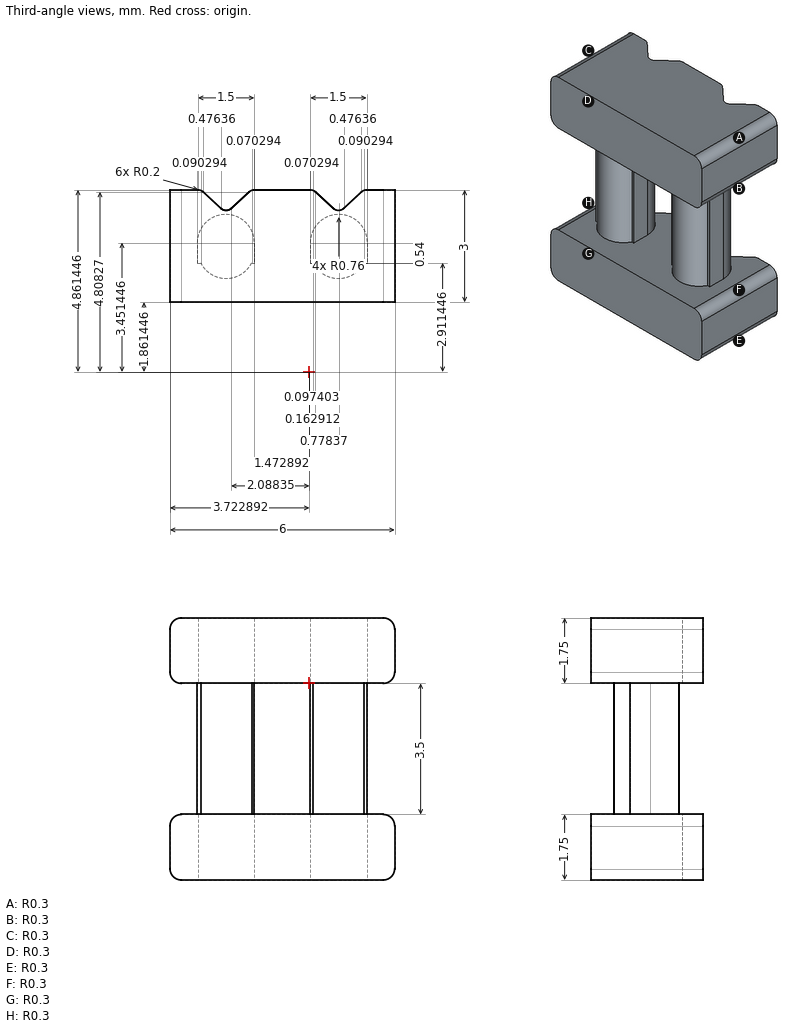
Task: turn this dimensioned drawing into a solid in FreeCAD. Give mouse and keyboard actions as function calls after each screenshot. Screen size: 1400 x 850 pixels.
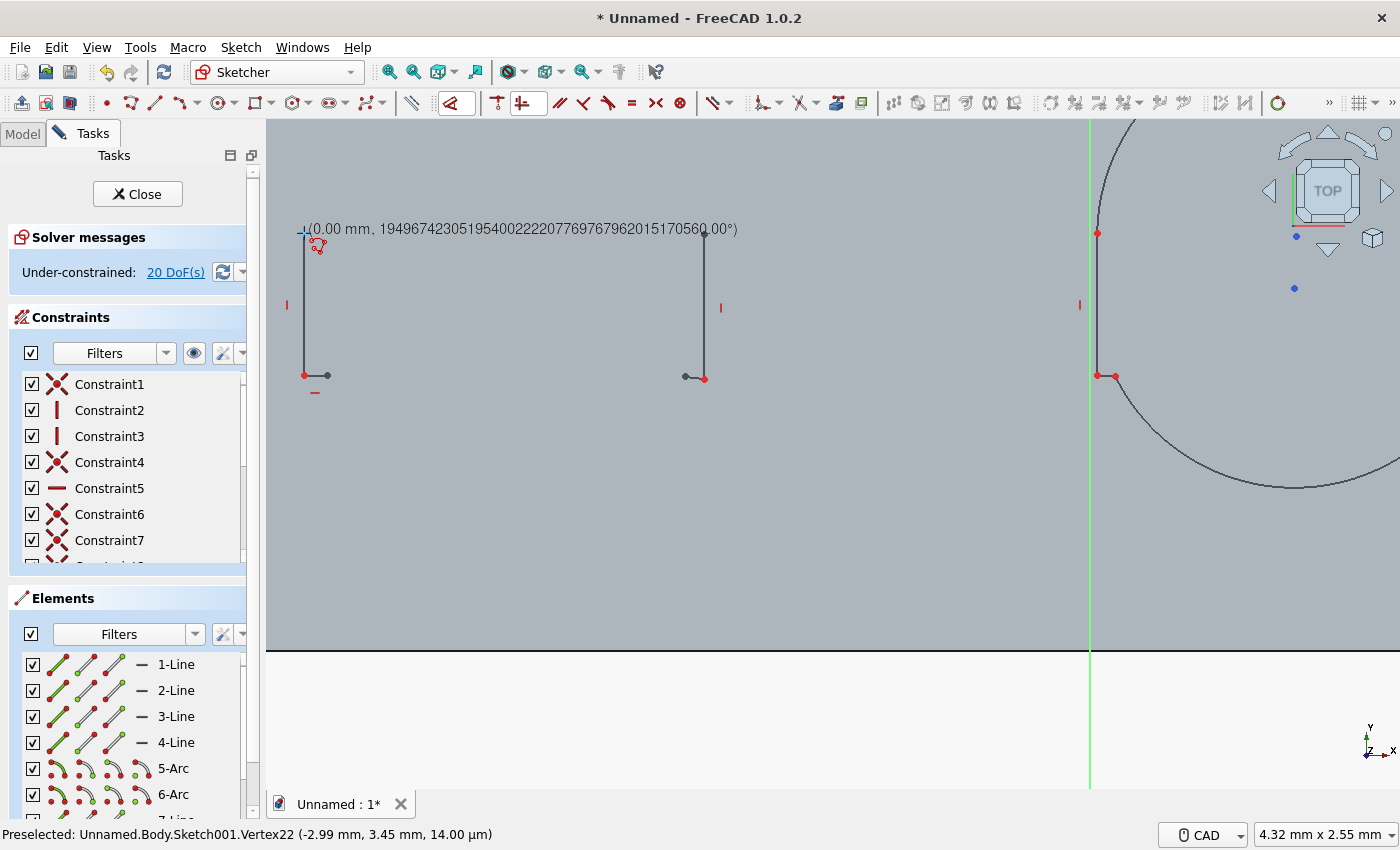
click(180, 104)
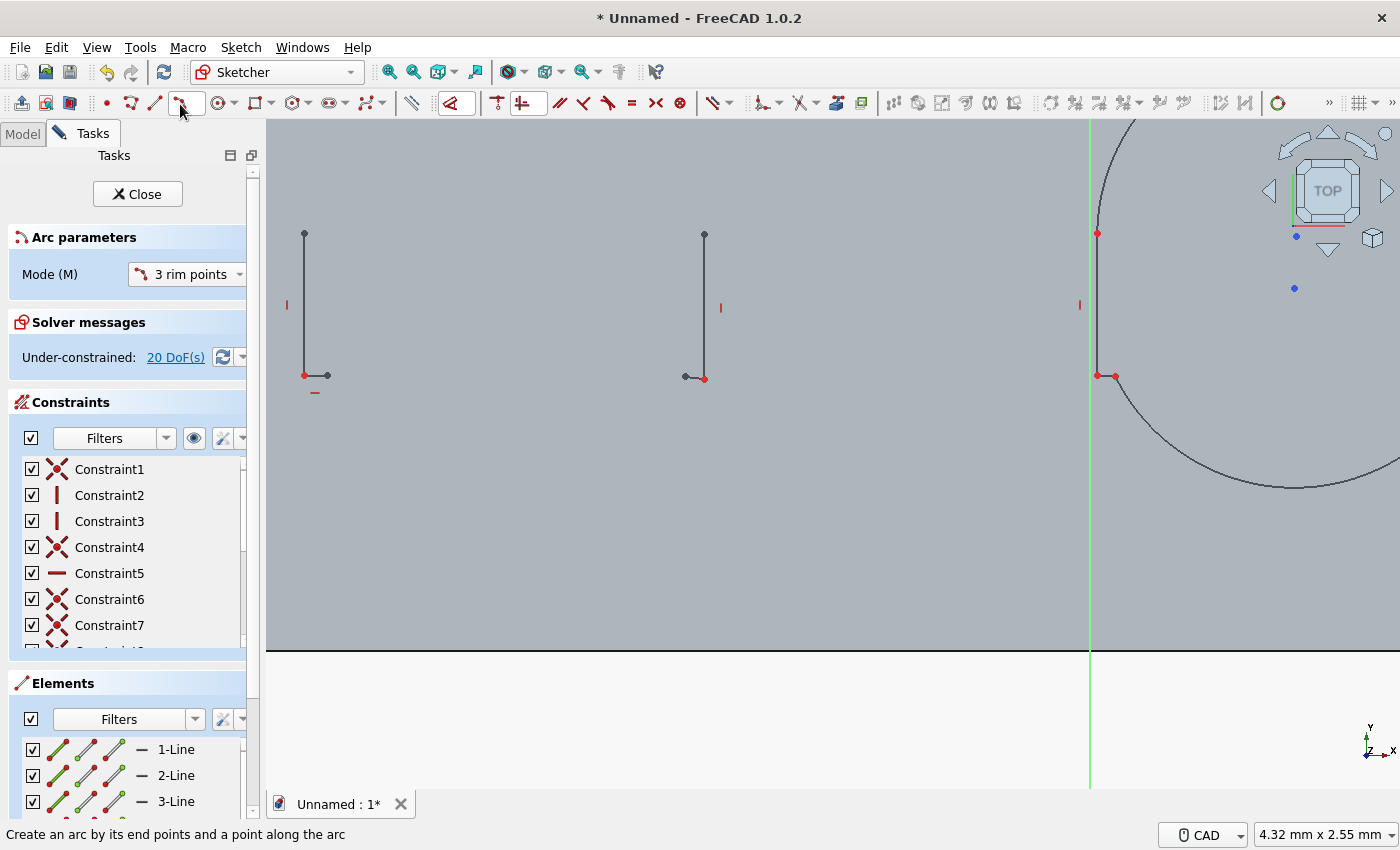
scroll(685, 375, up, 3)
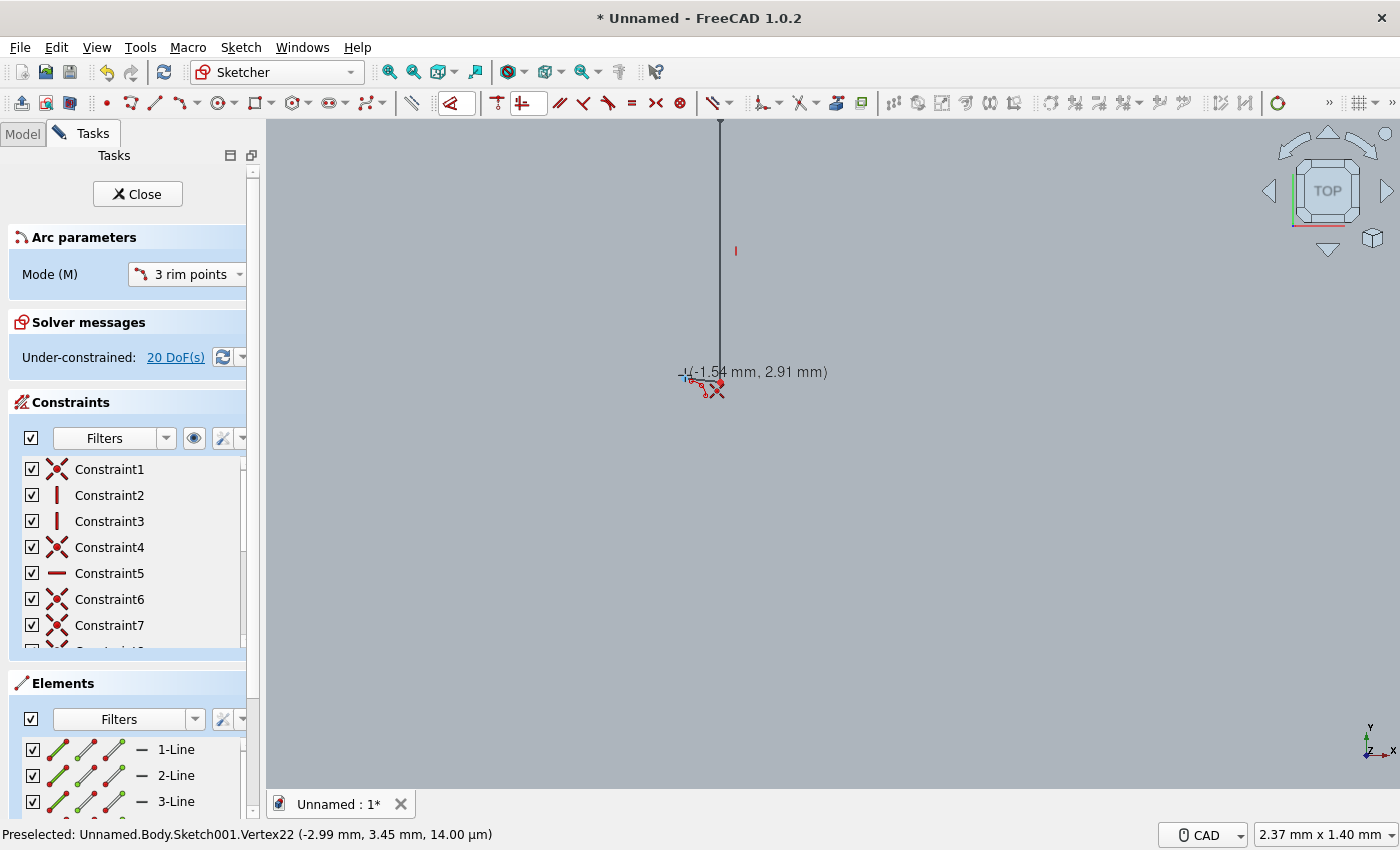
click(685, 378)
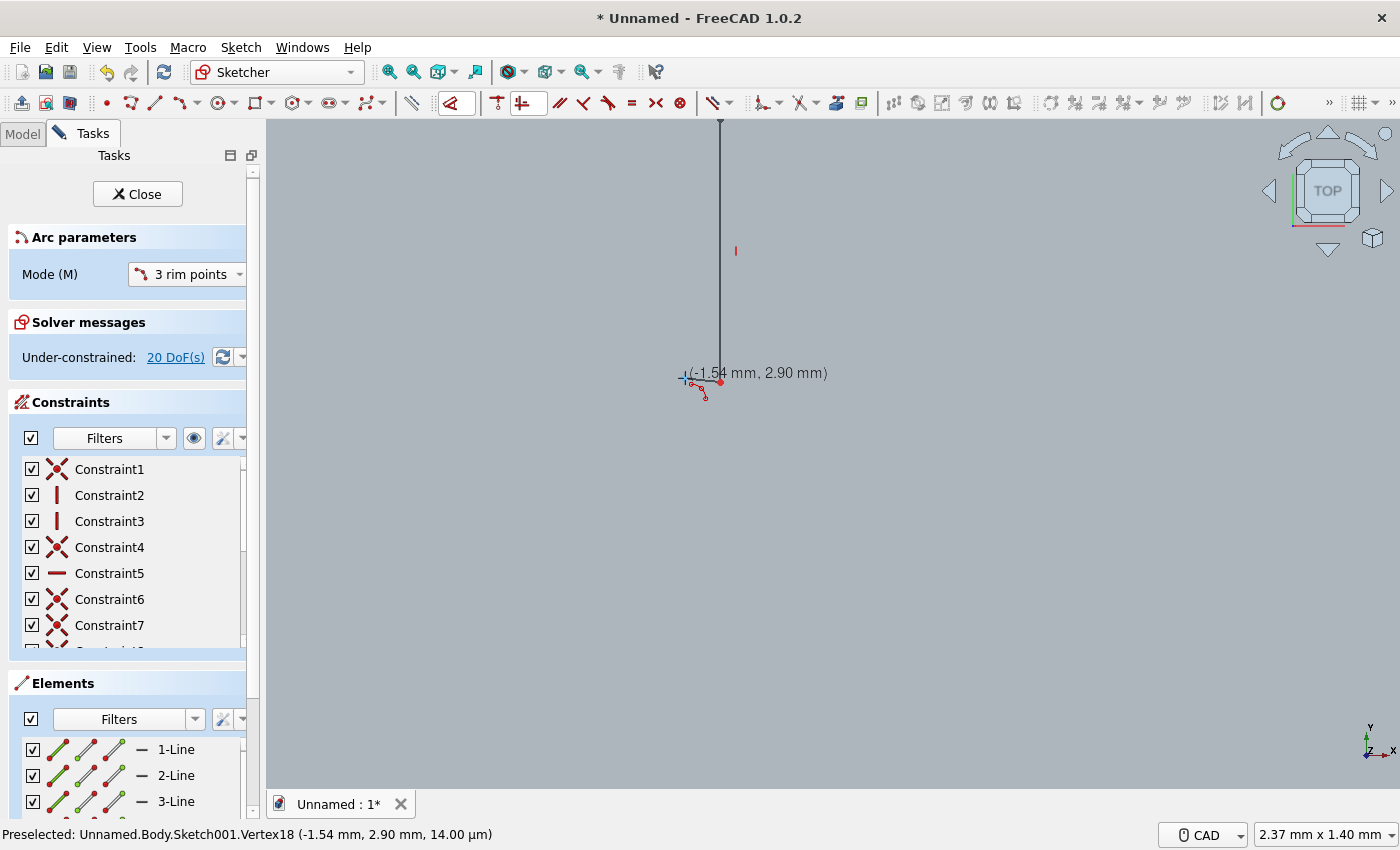
scroll(685, 376, down, 8)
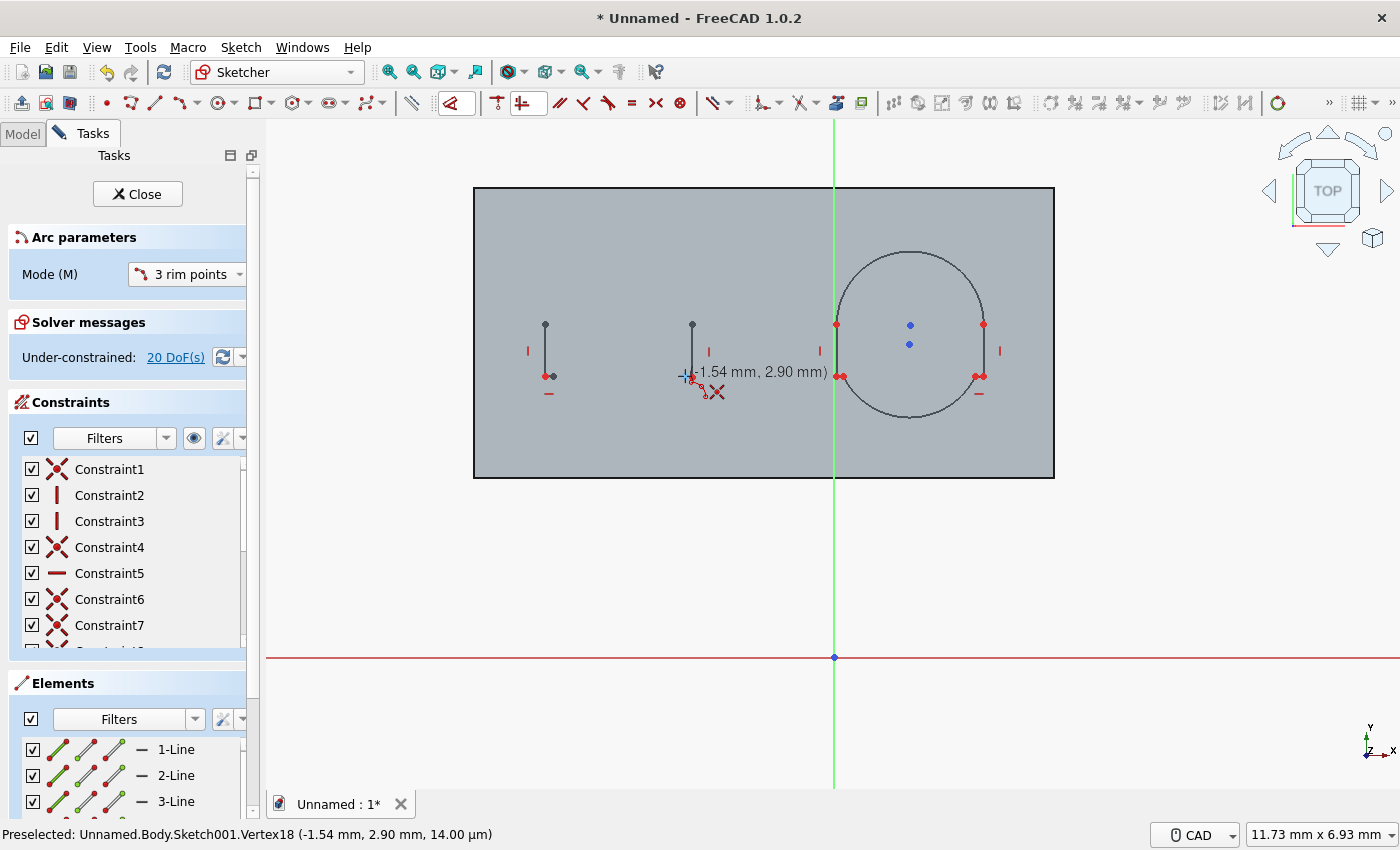
scroll(554, 376, up, 7)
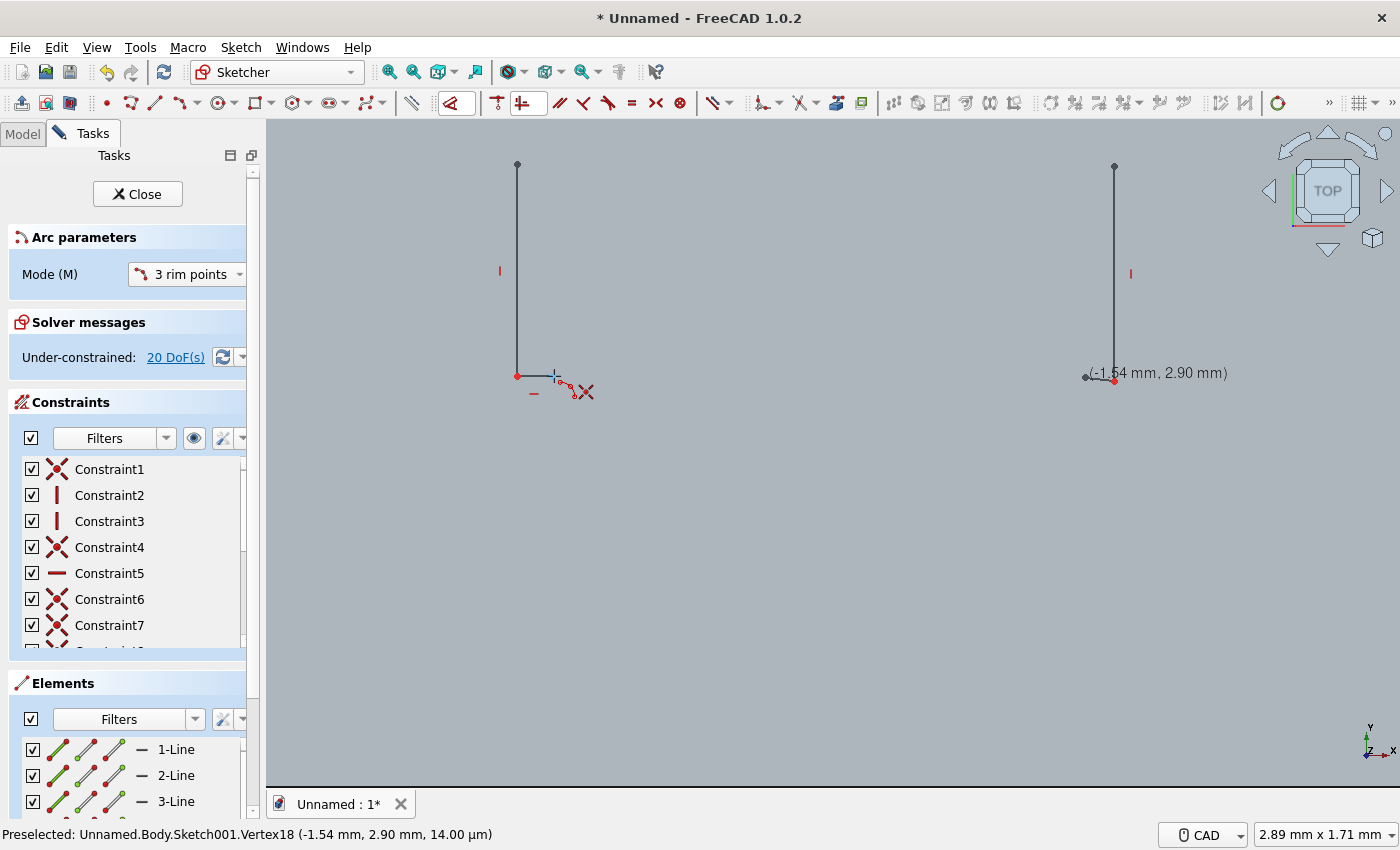
click(553, 376)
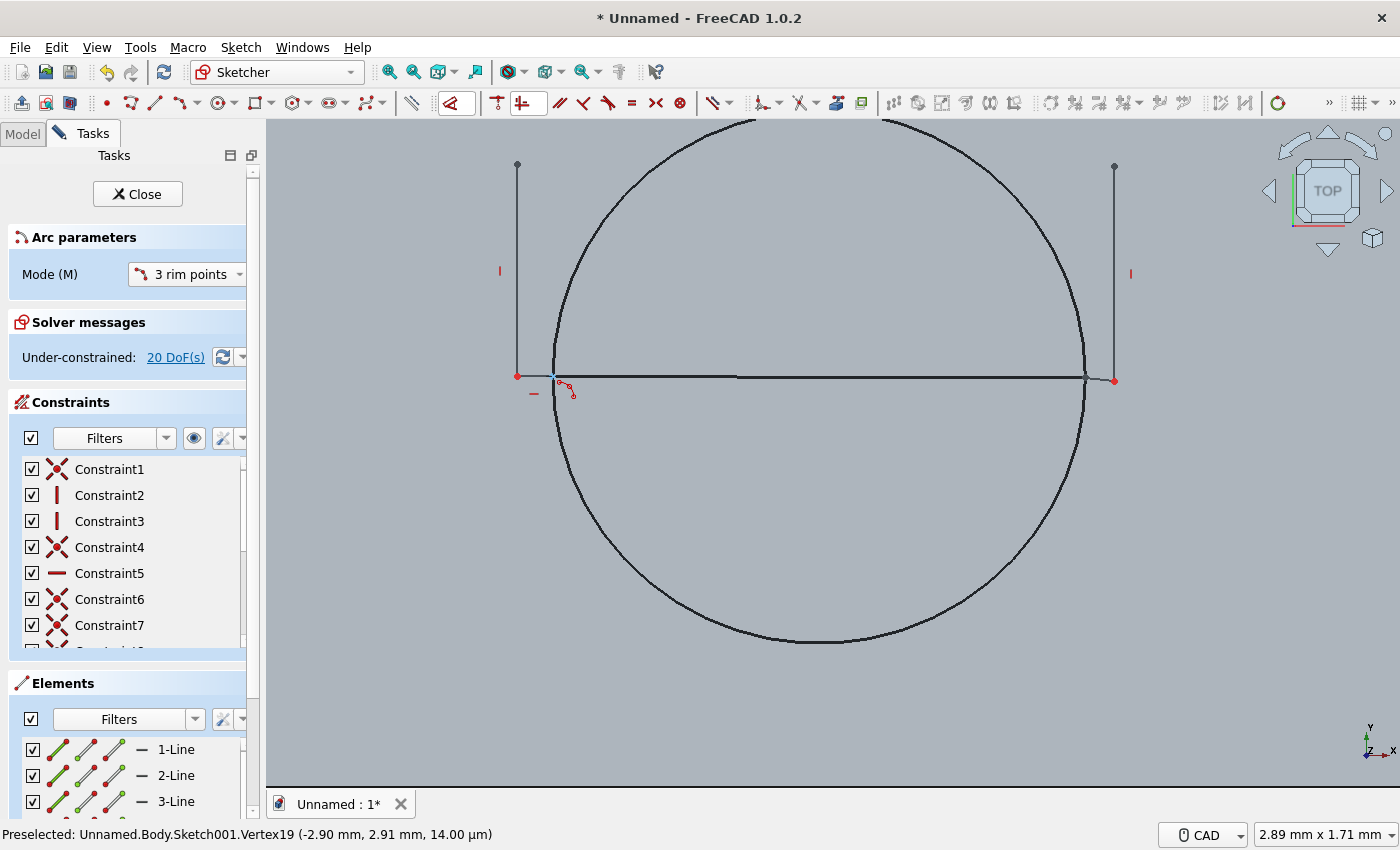
scroll(554, 376, down, 7)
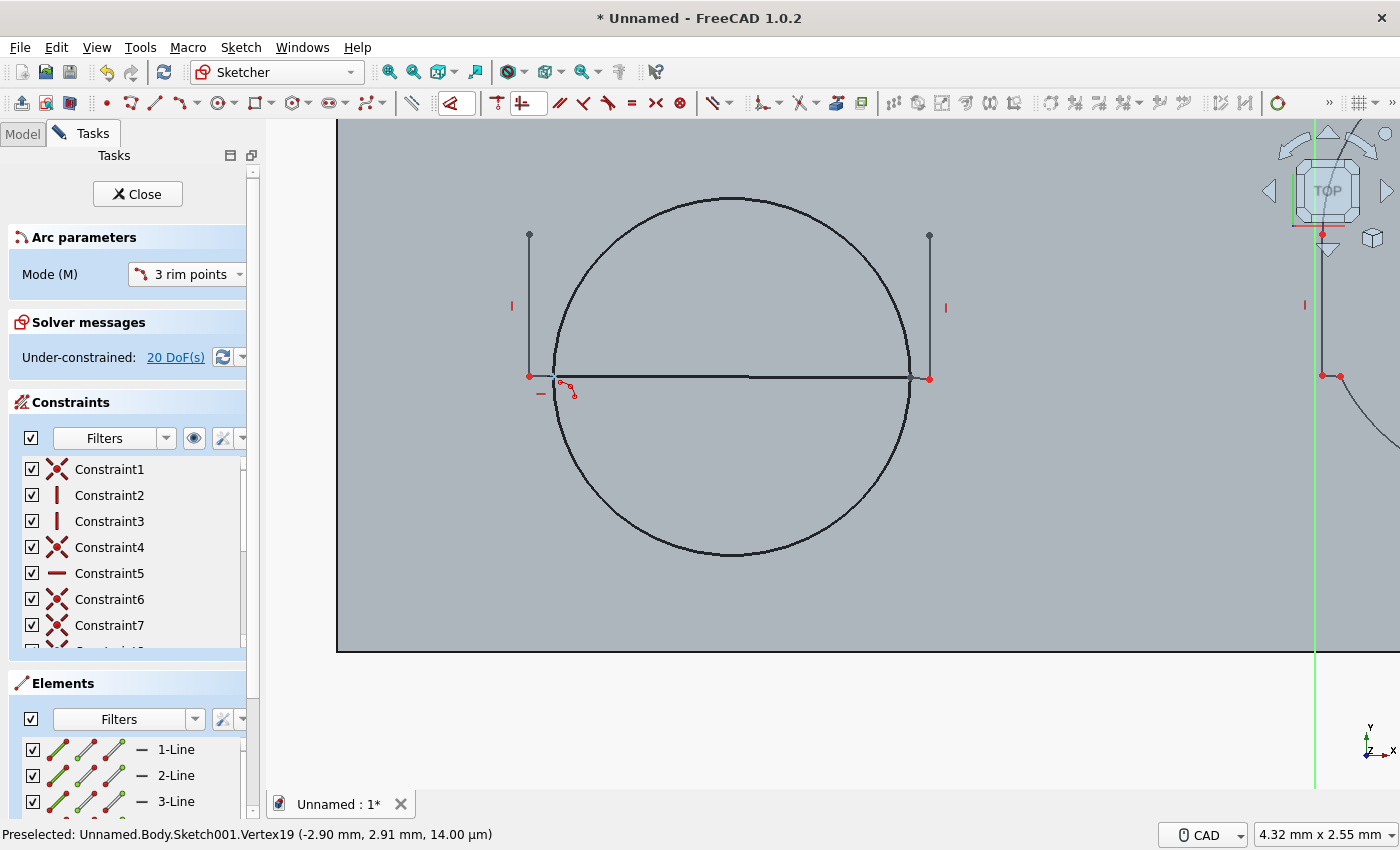
click(619, 417)